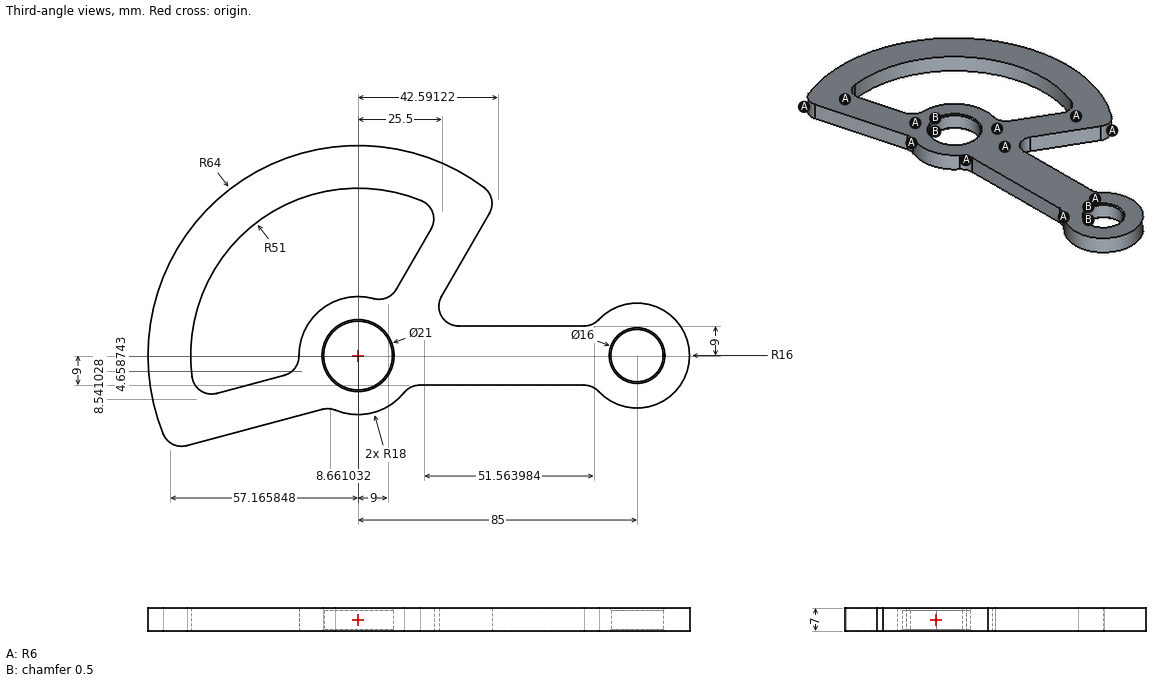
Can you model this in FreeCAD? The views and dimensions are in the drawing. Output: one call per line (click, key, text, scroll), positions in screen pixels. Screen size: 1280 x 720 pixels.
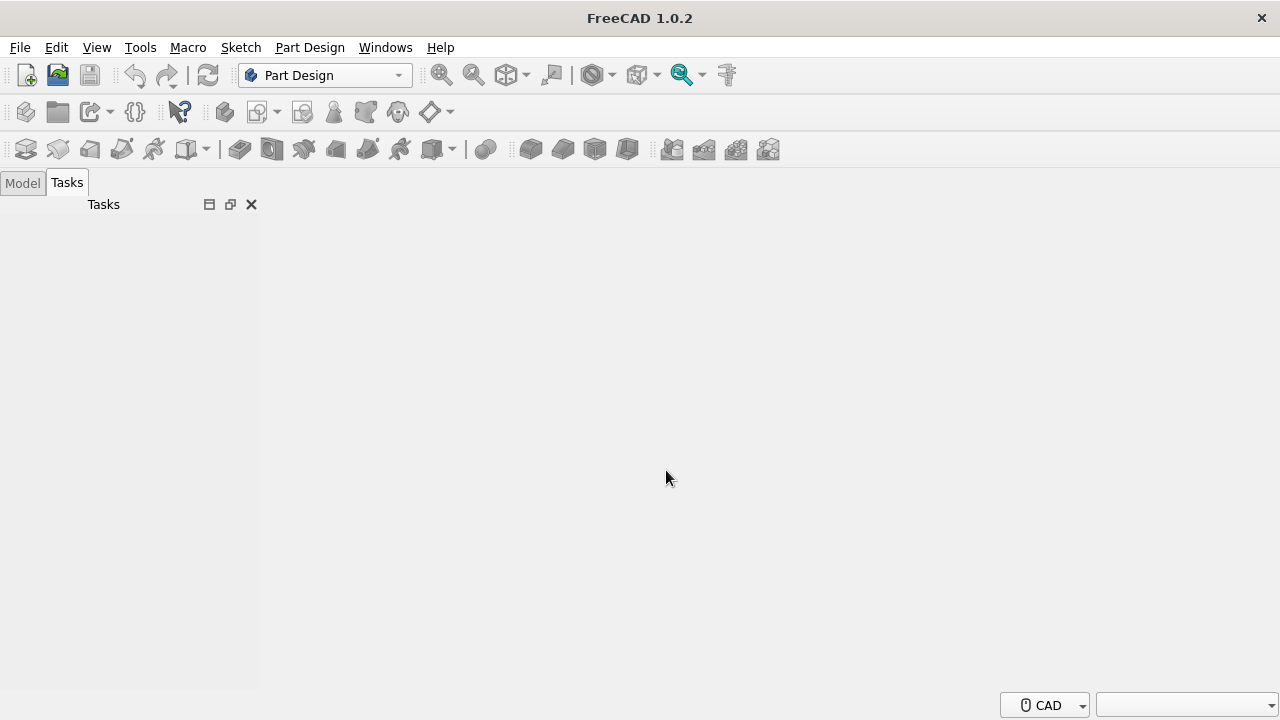
key(ctrl+n)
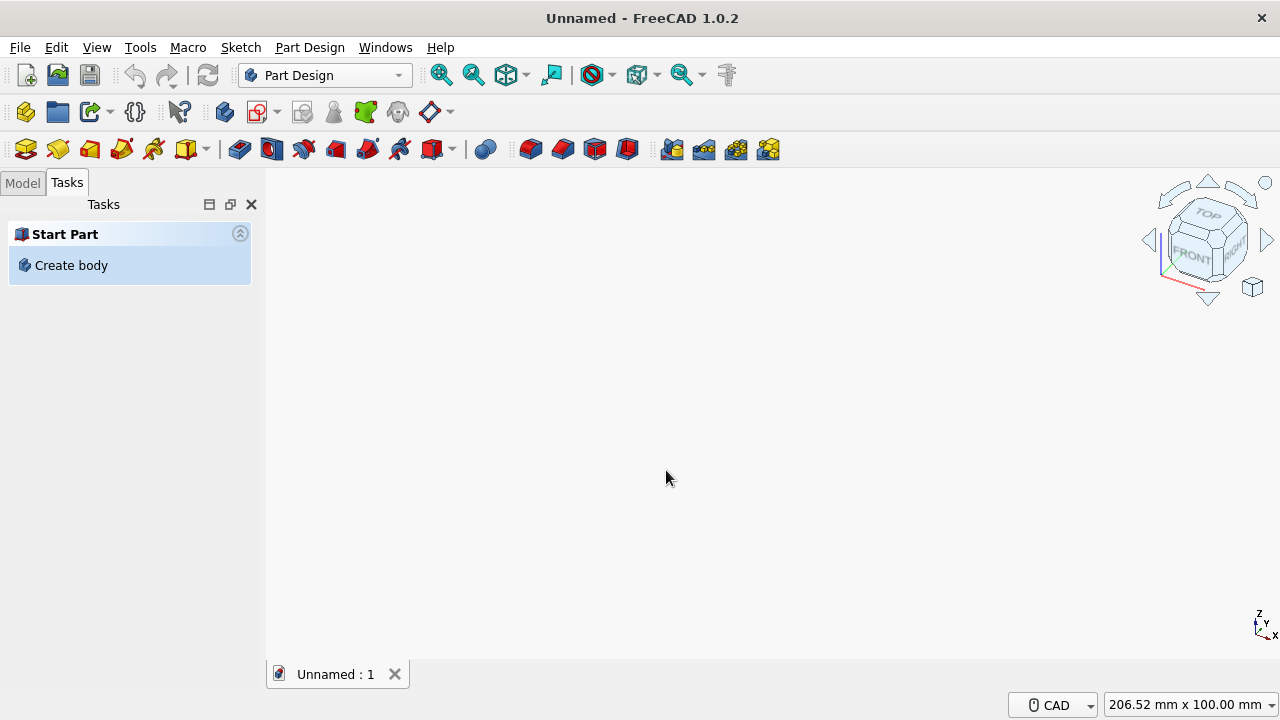
click(258, 112)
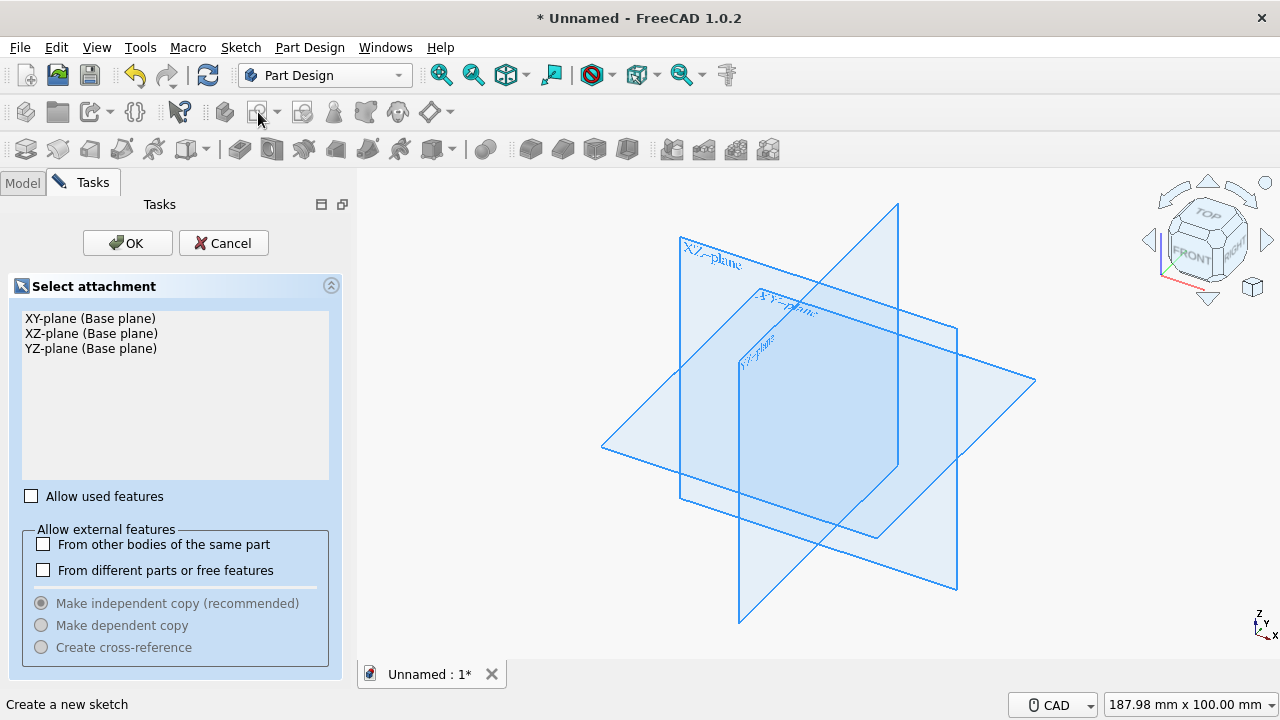
click(82, 318)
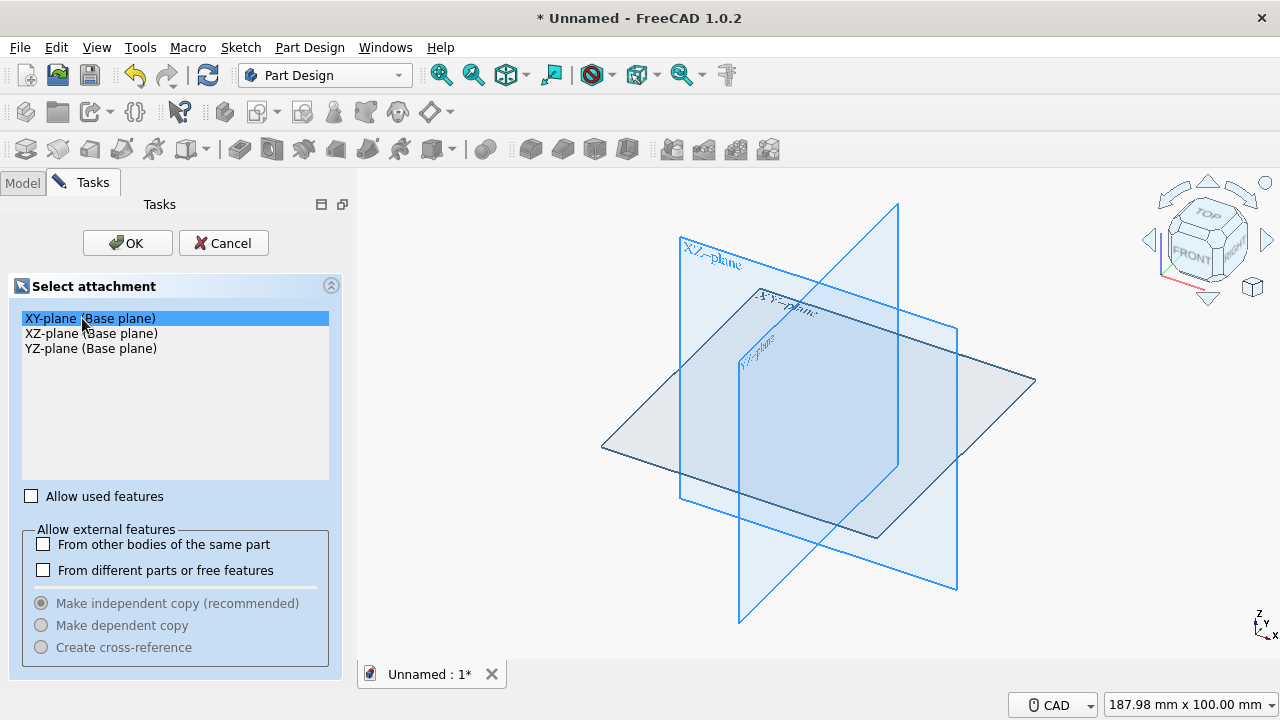
click(128, 243)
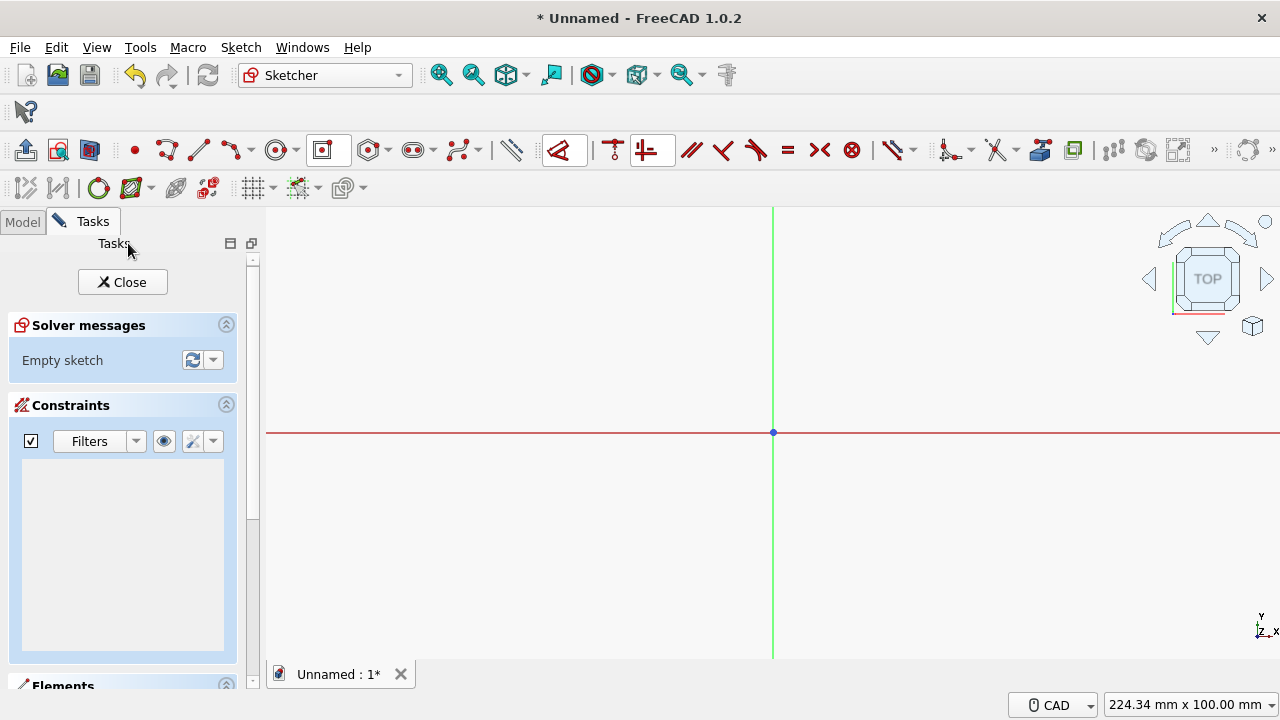
scroll(294, 631, down, 1)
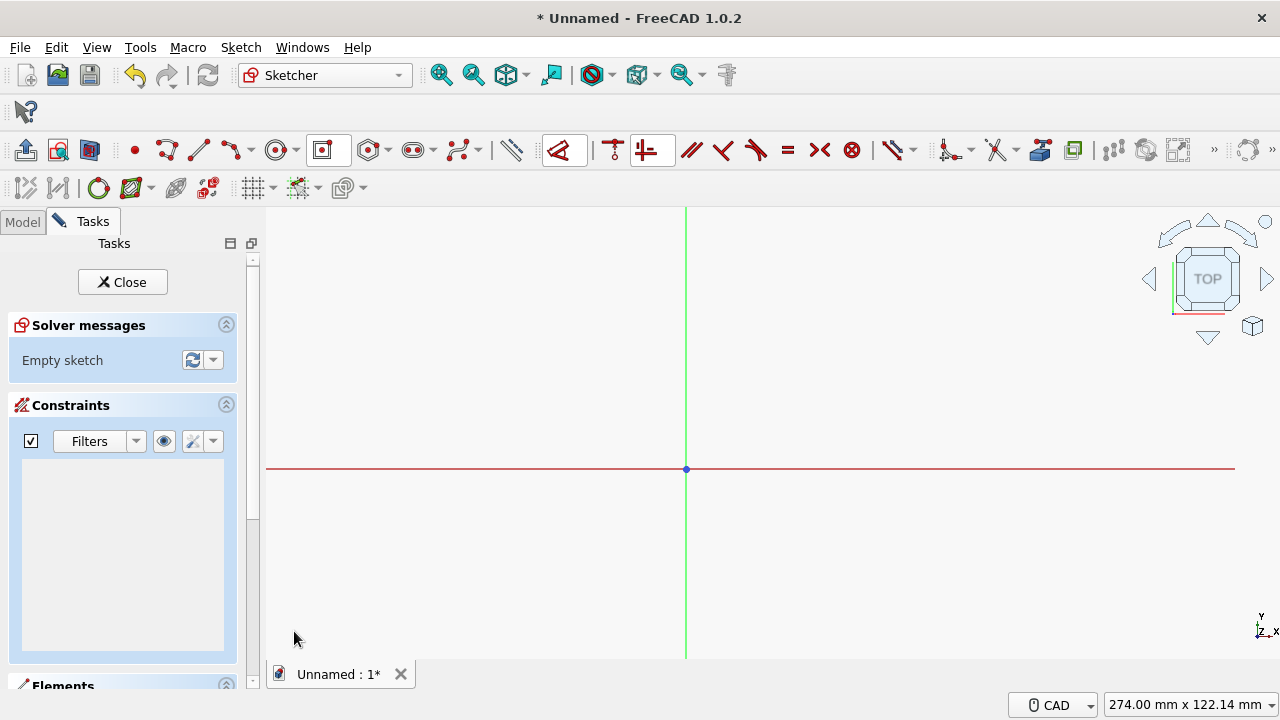
click(168, 150)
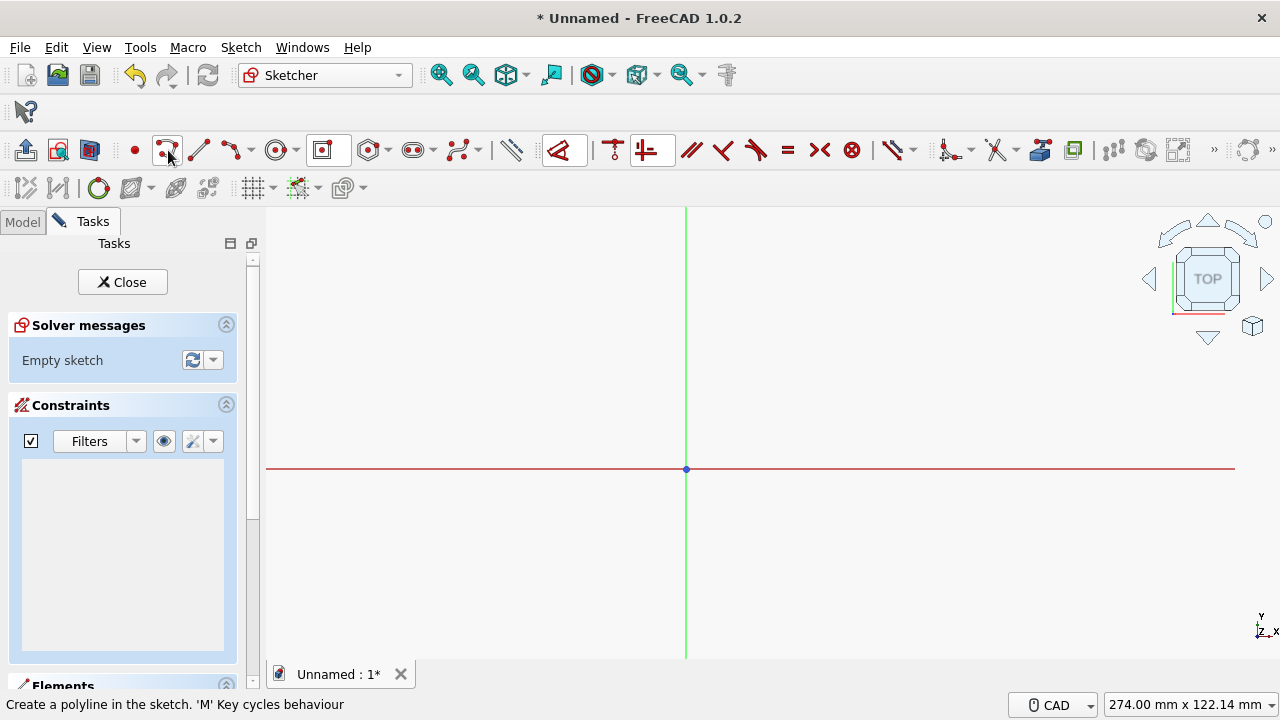
click(952, 436)
click(761, 436)
click(844, 292)
right_click(844, 292)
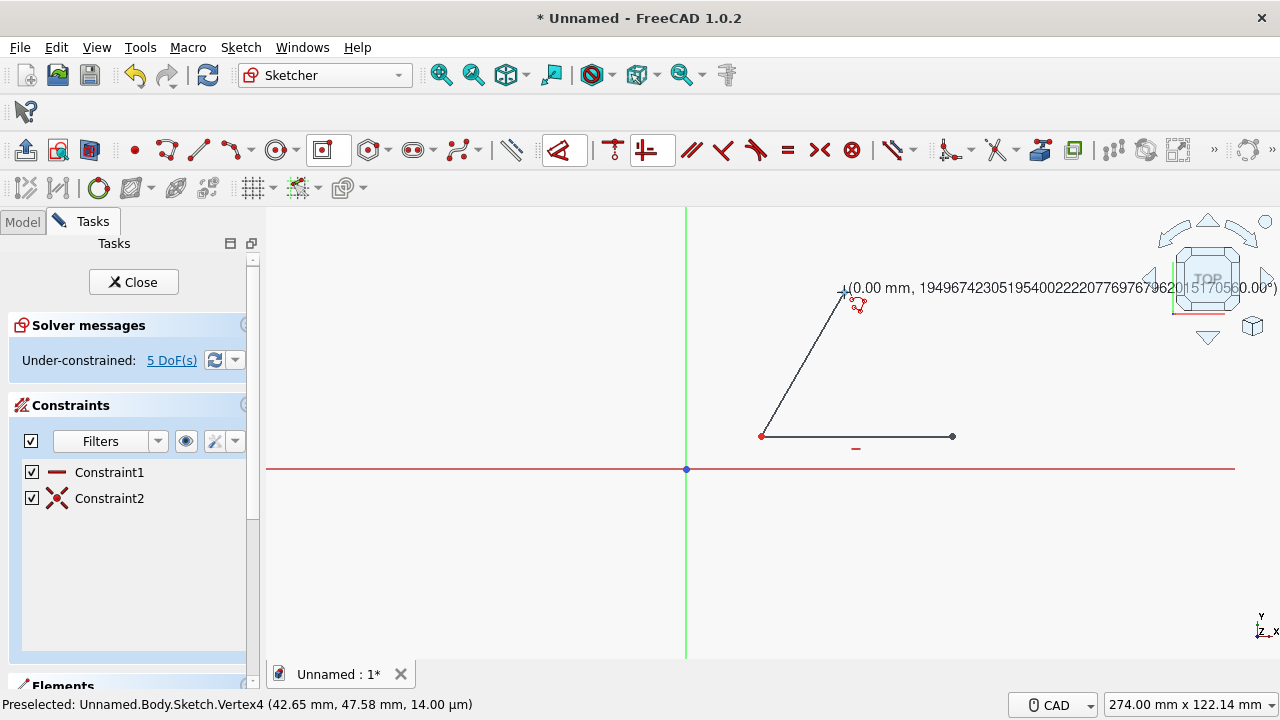
click(200, 150)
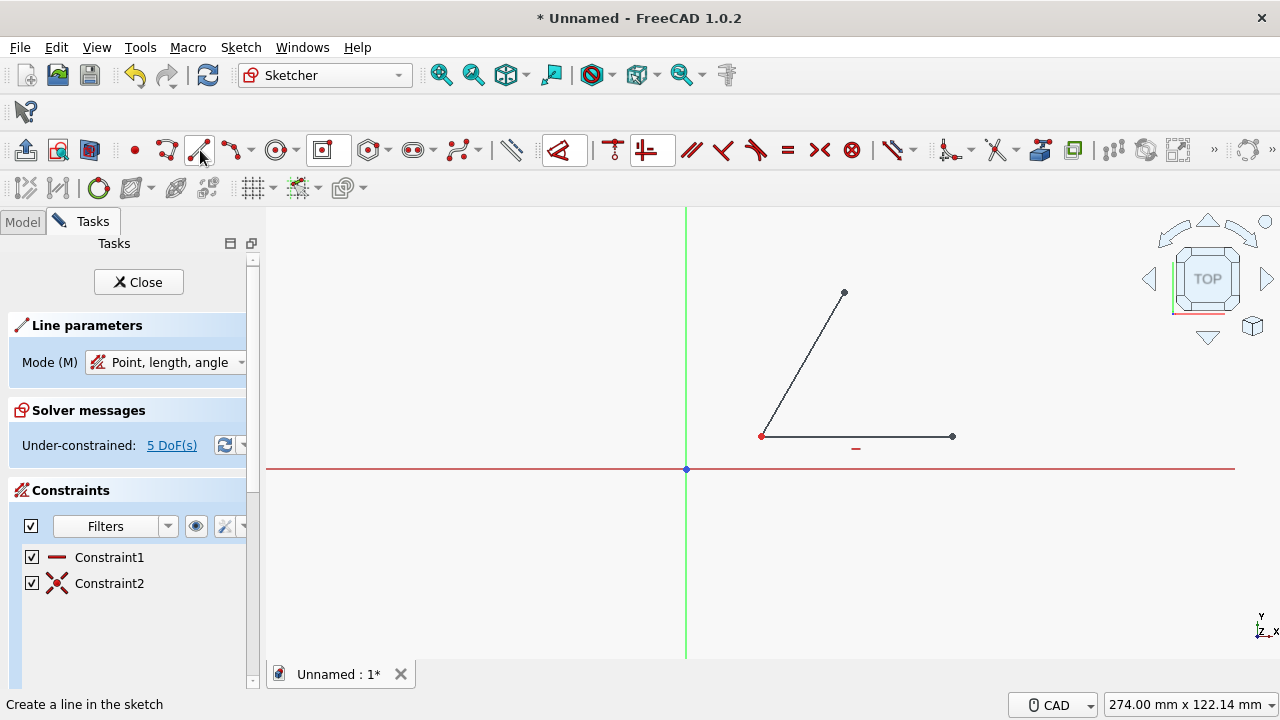
click(475, 576)
click(654, 527)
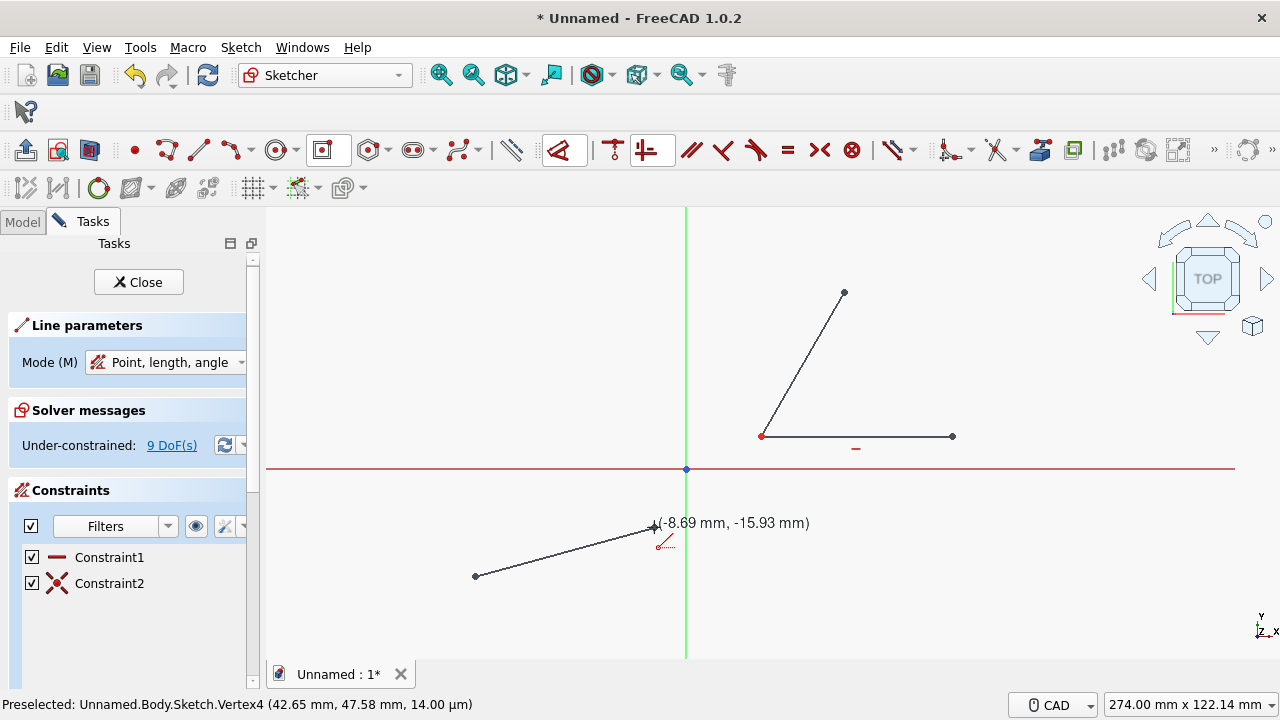
click(744, 502)
click(952, 502)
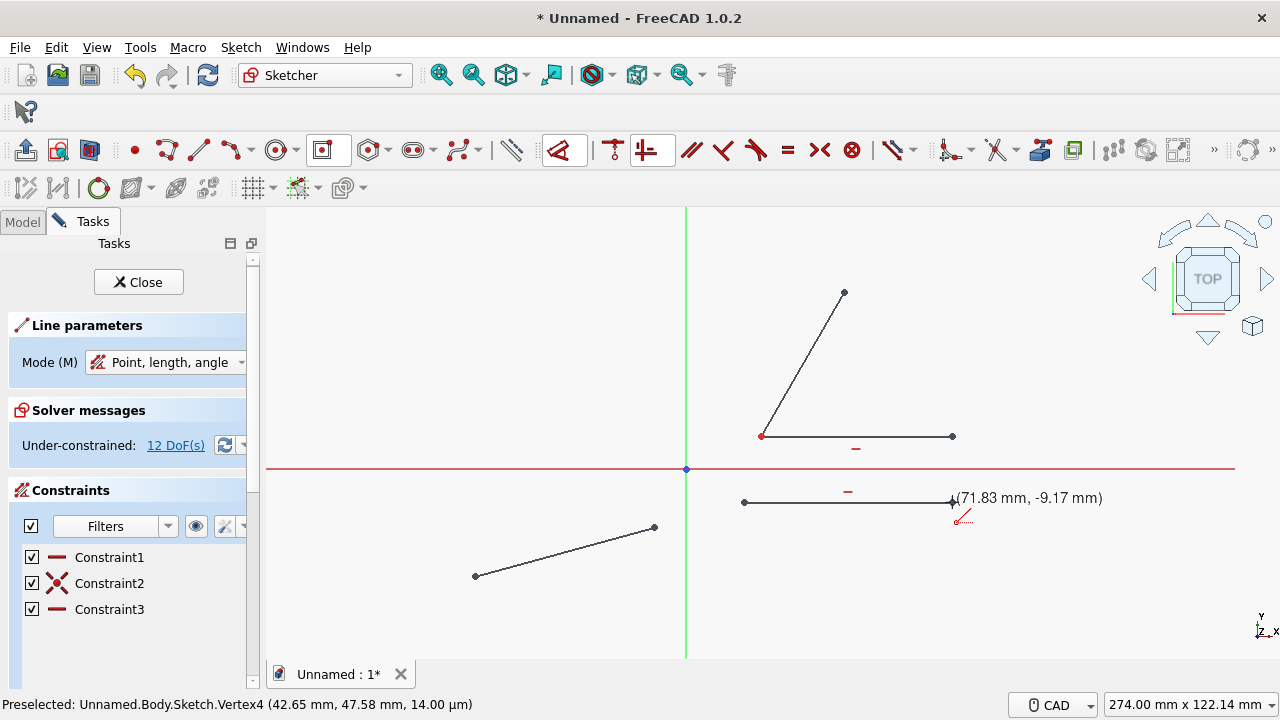
click(232, 150)